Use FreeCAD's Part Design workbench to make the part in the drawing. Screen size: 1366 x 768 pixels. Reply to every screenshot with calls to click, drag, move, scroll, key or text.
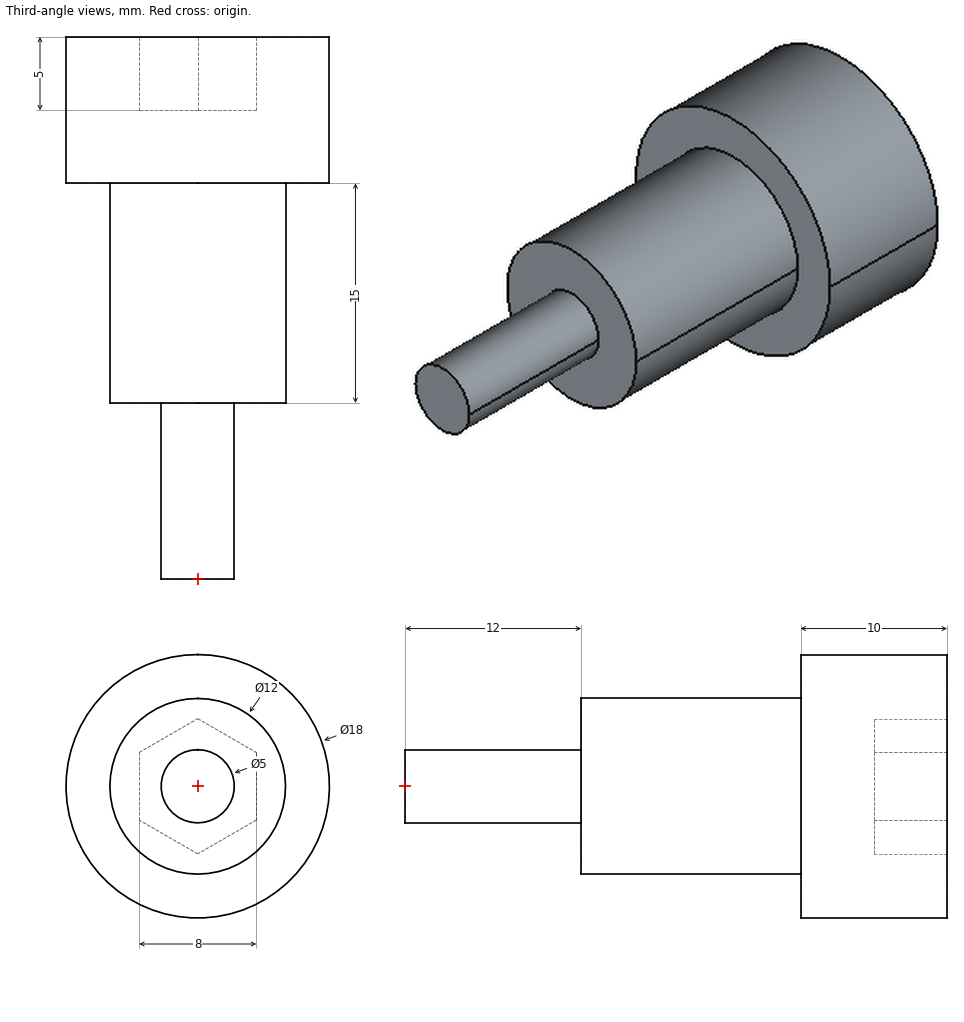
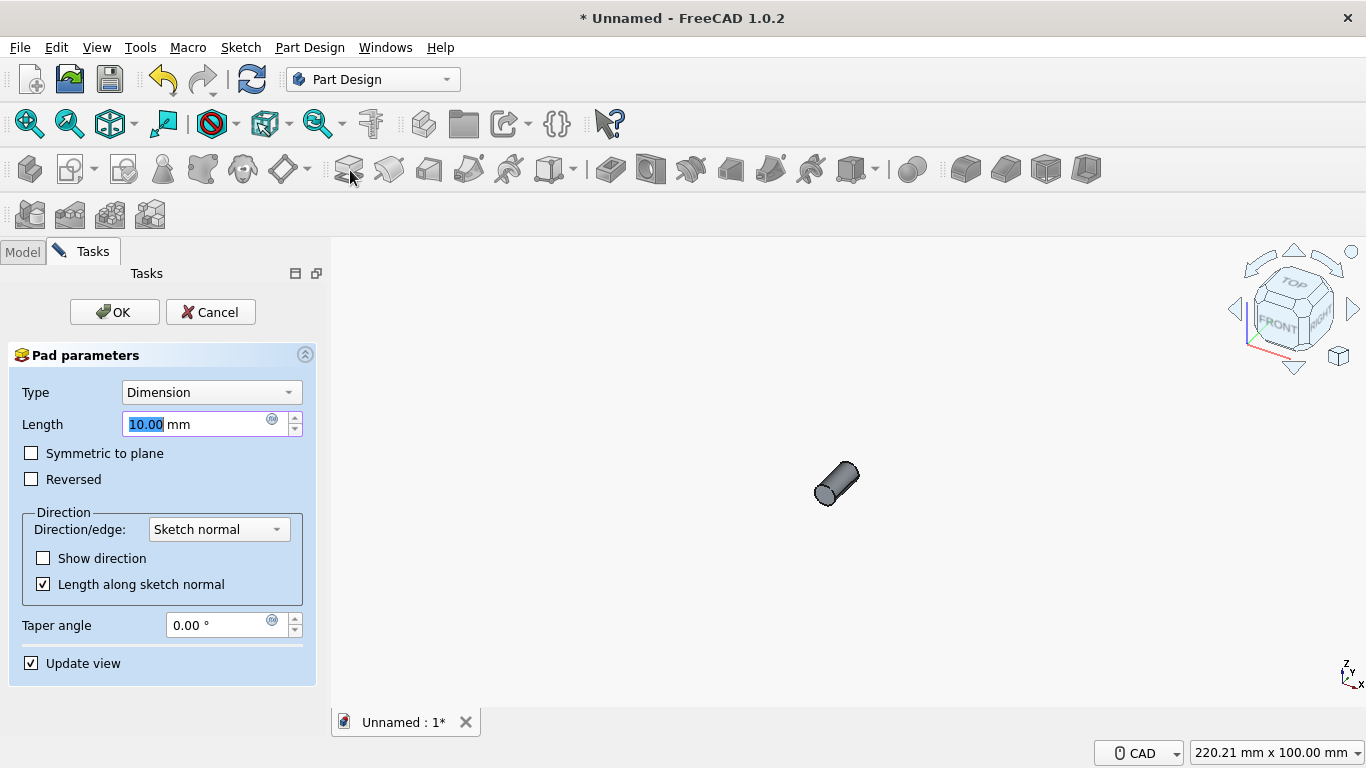
text(12)
key(Tab)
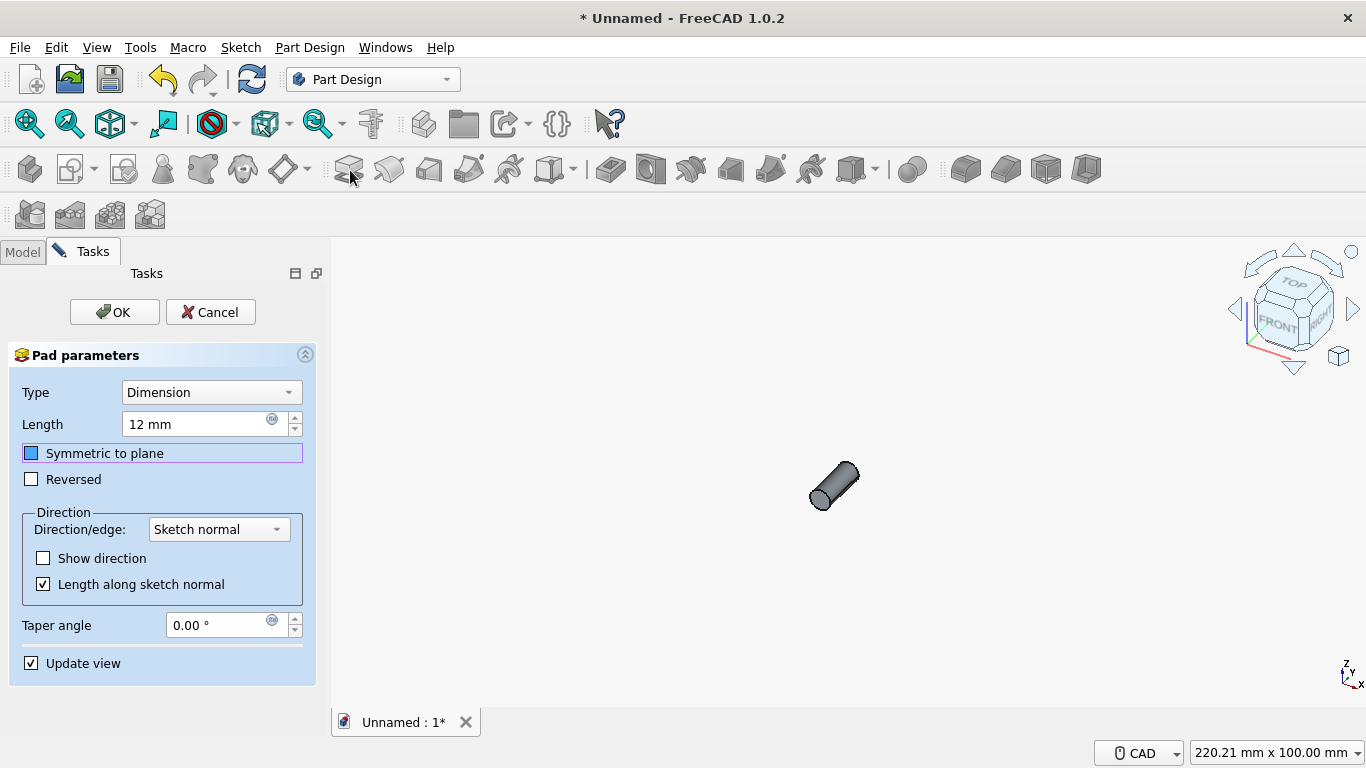
click(30, 479)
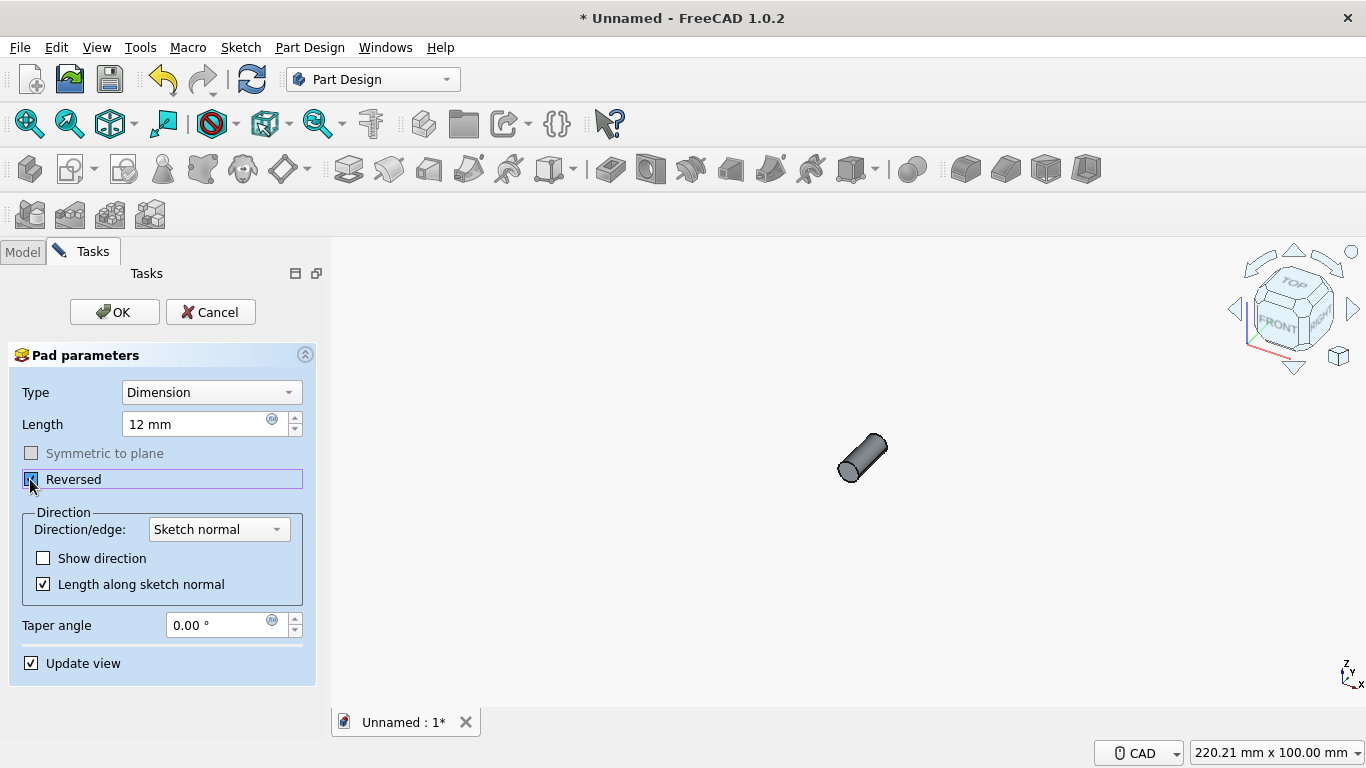
click(115, 312)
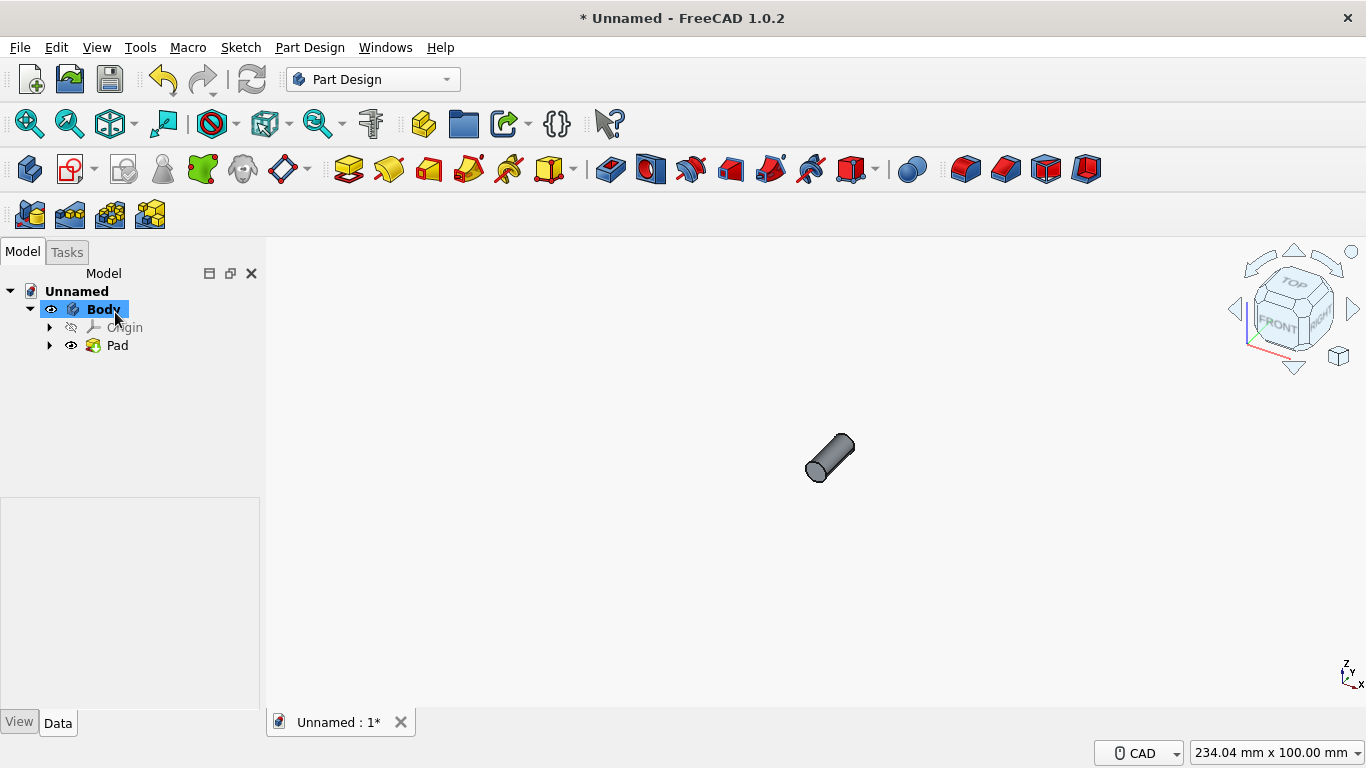
click(30, 124)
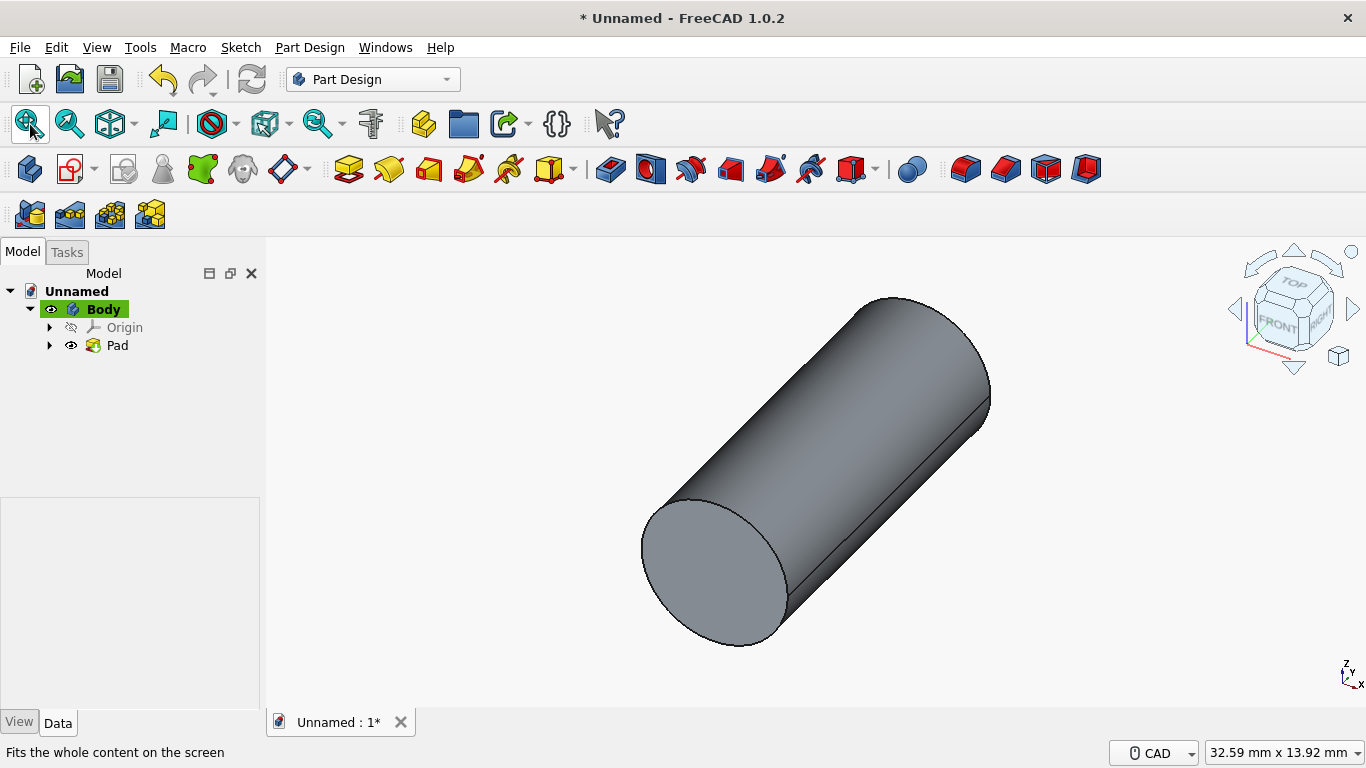
key(4)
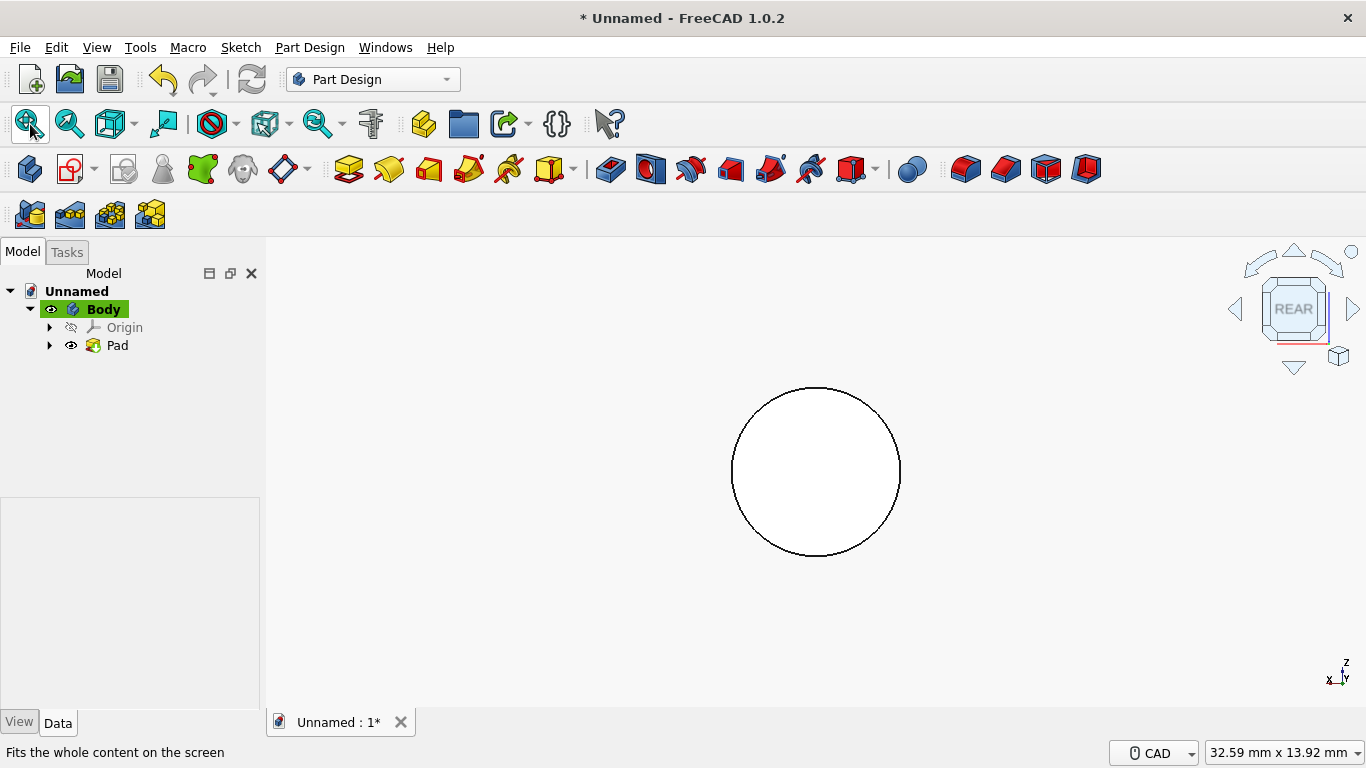
click(30, 124)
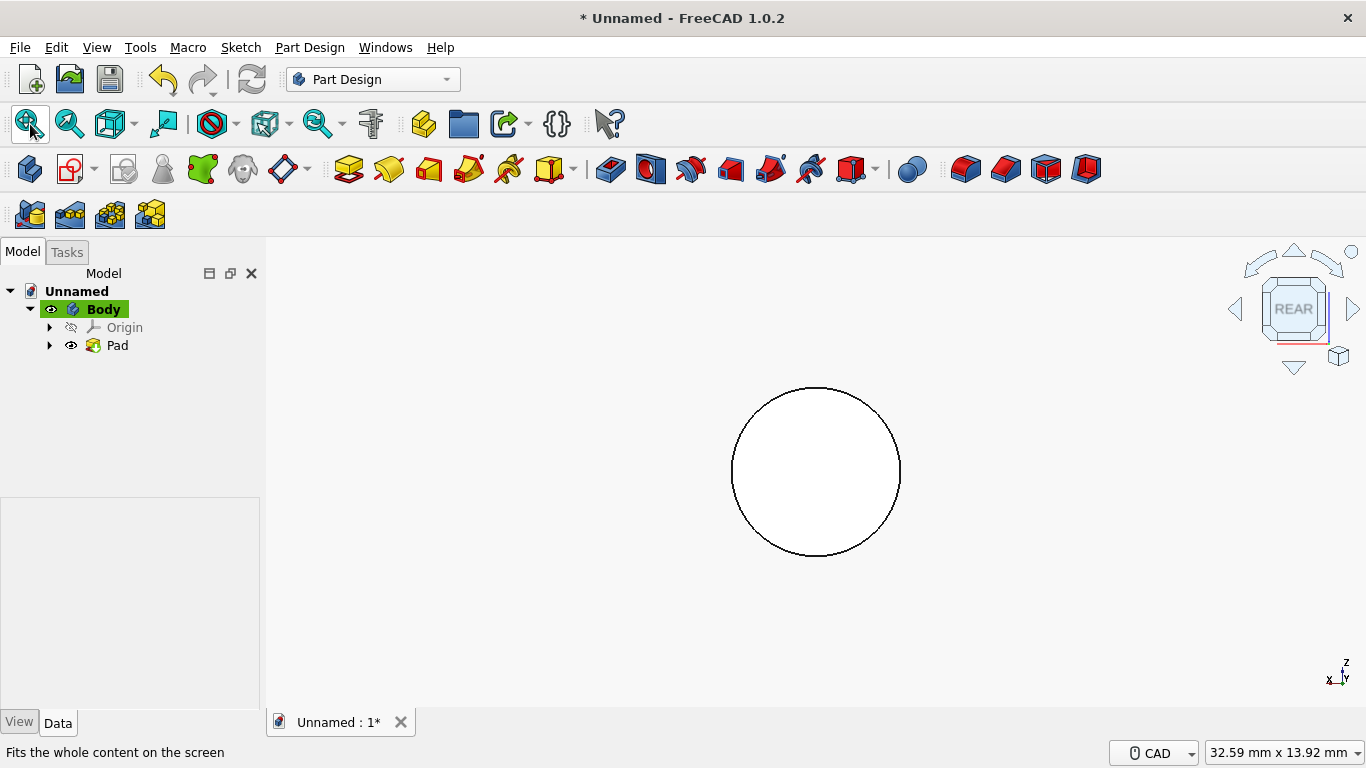
click(816, 471)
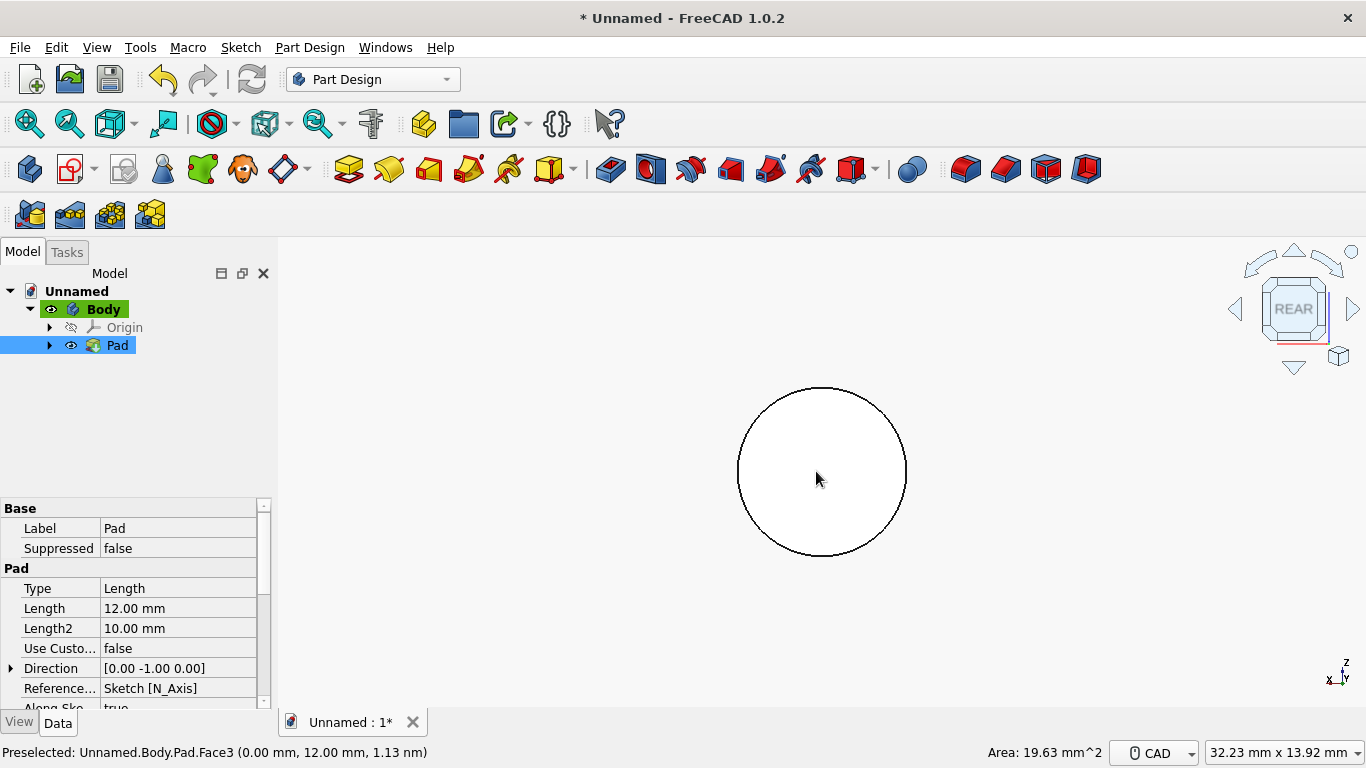
click(70, 170)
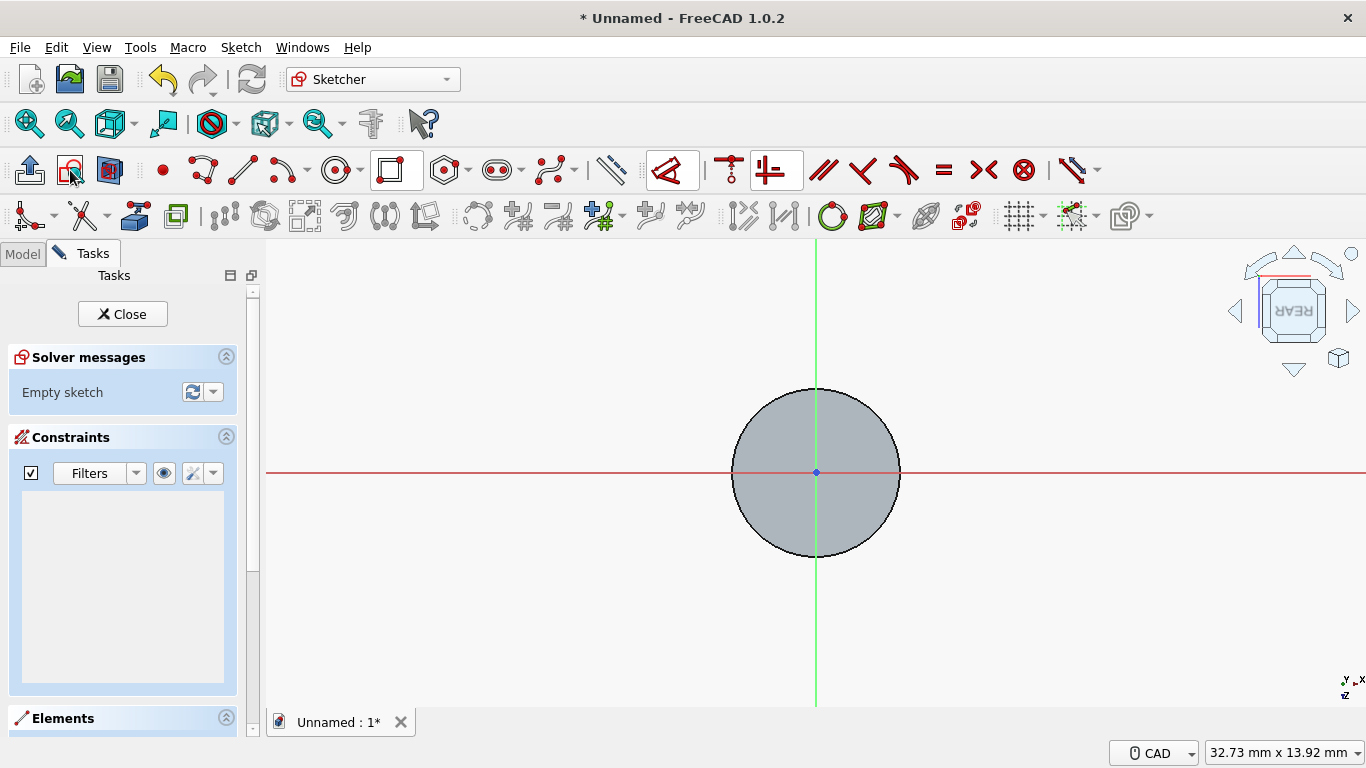
scroll(608, 473, down, 2)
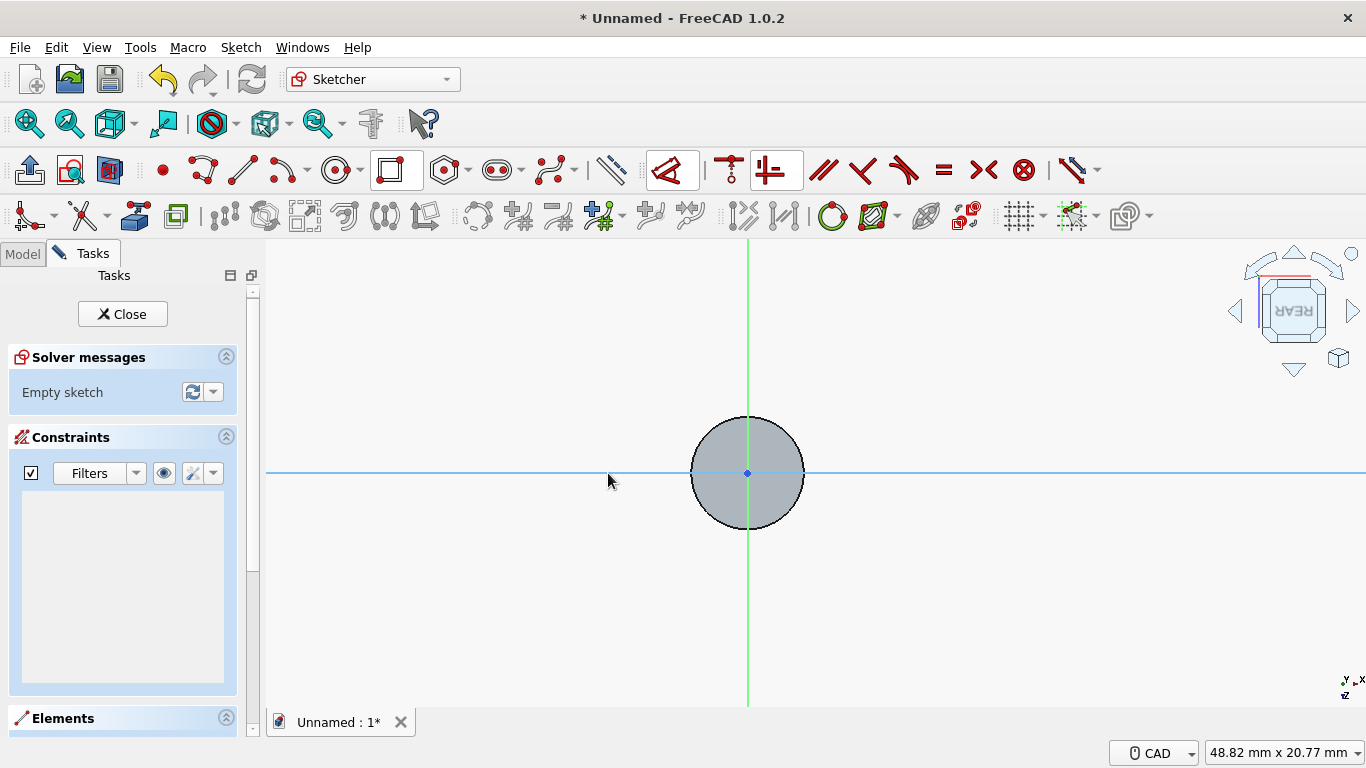
click(336, 170)